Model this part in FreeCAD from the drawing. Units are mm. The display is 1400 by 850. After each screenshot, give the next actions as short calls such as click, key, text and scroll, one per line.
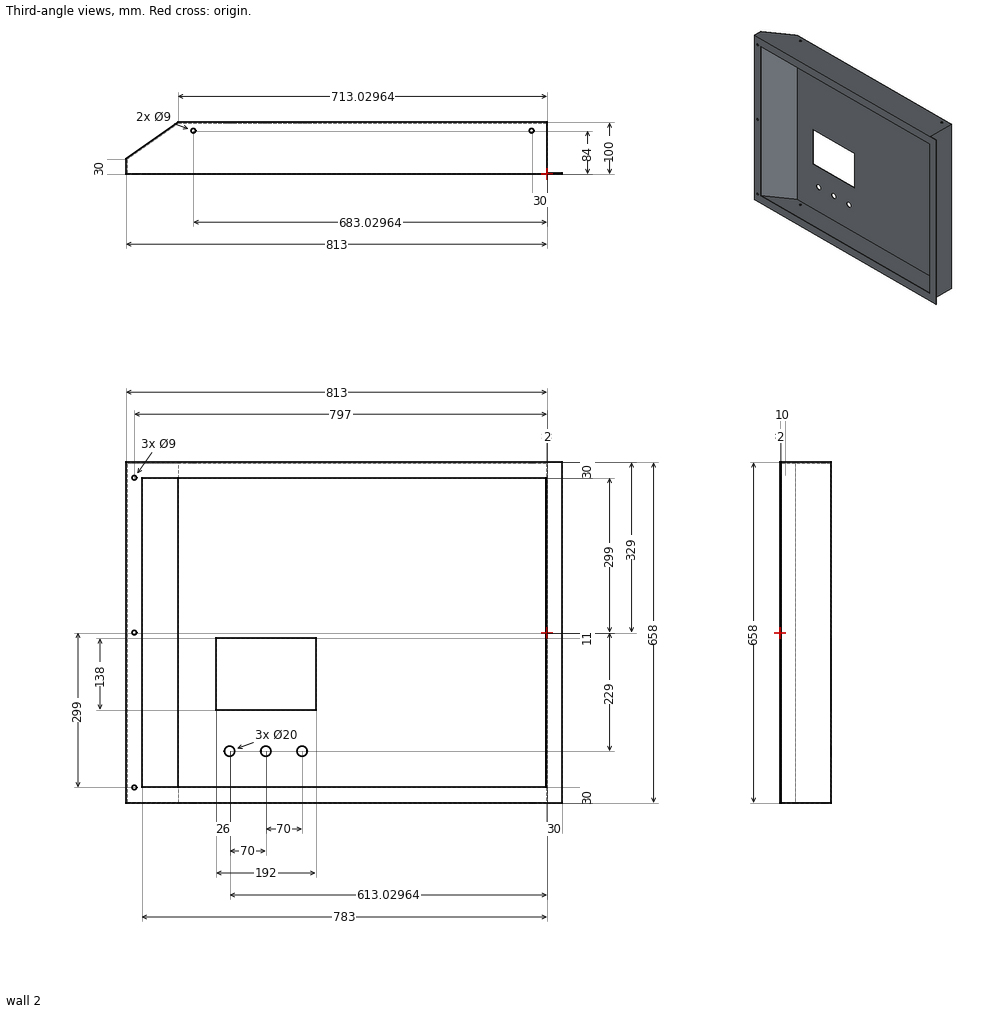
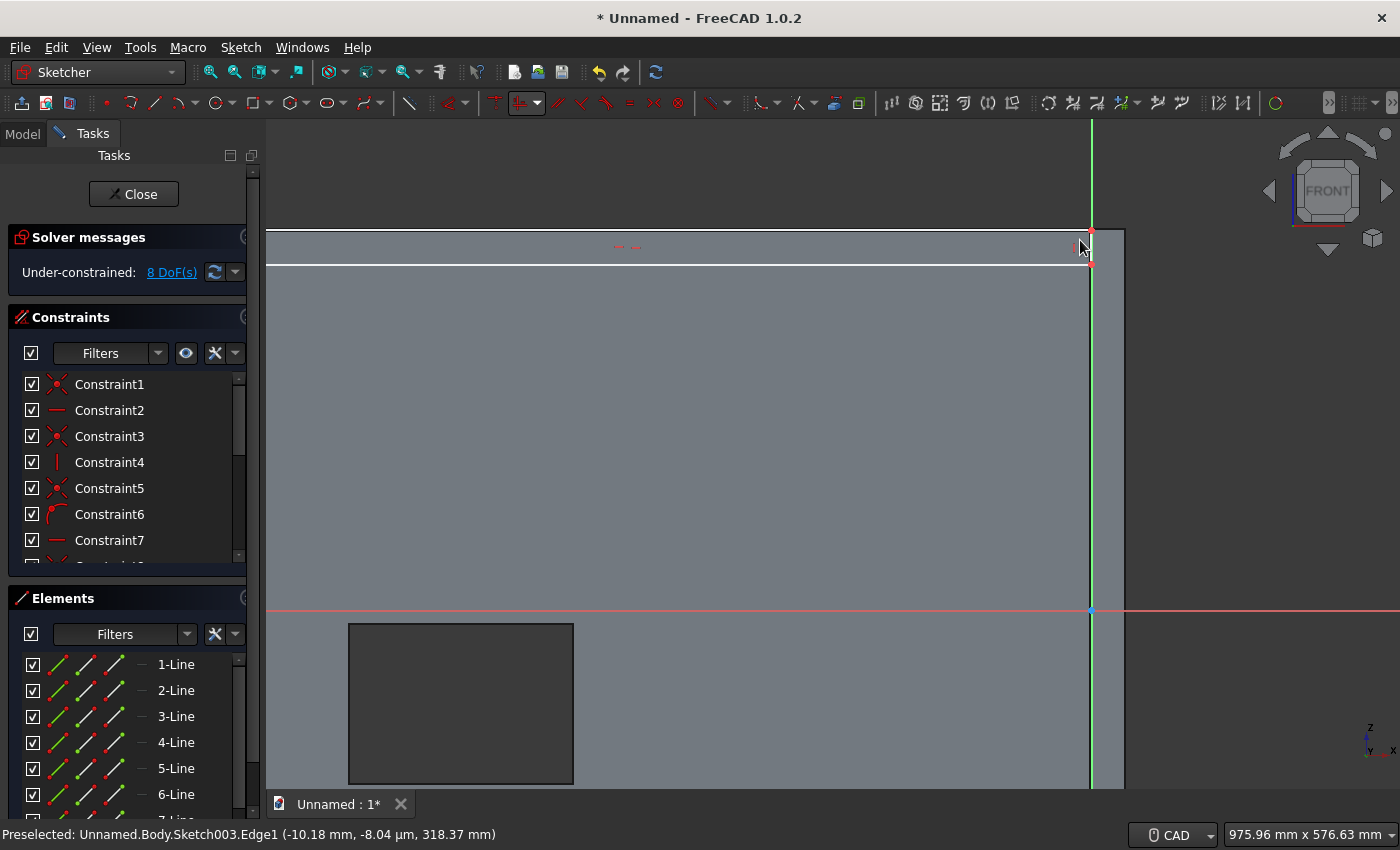
scroll(941, 263, down, 3)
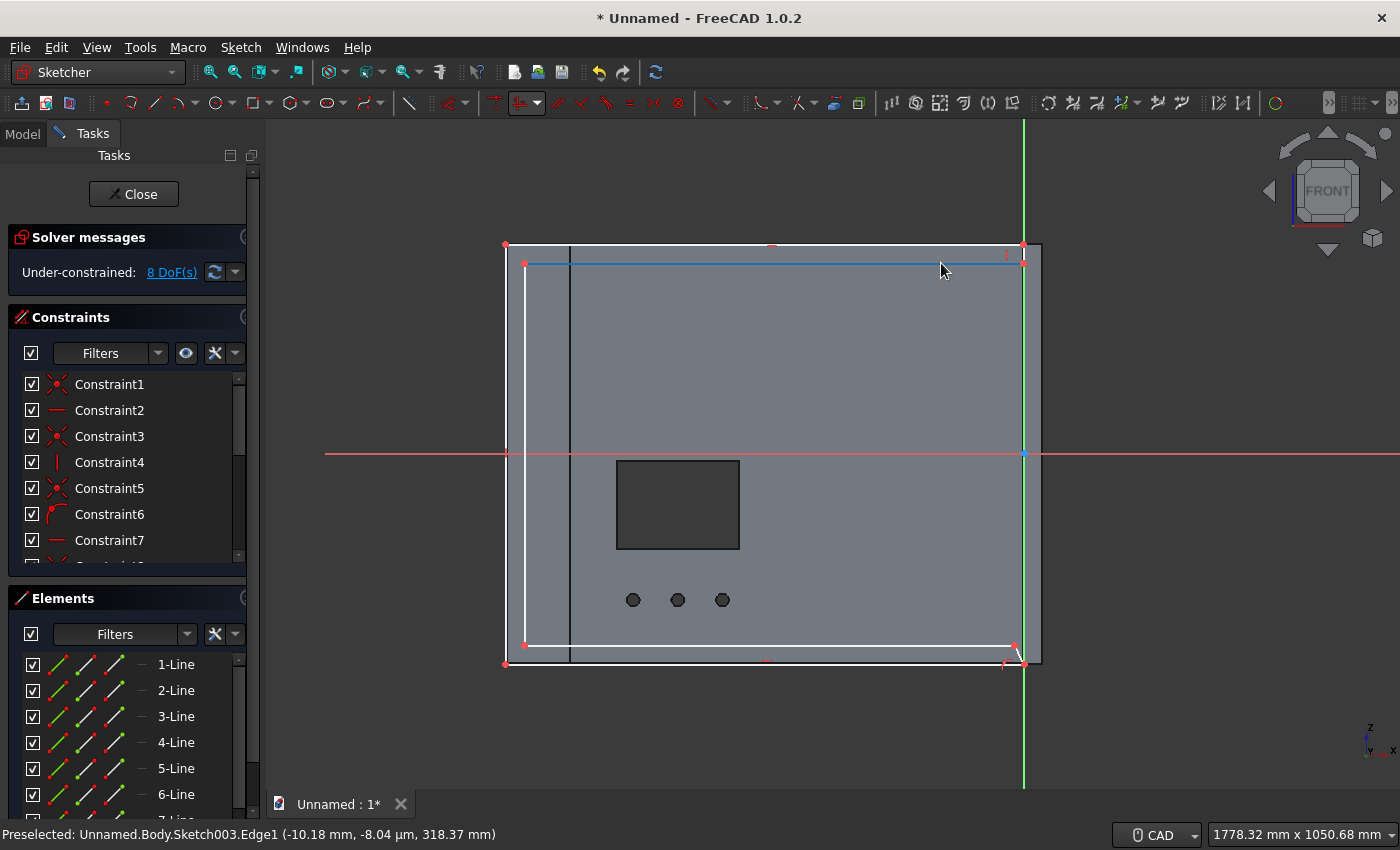
scroll(1018, 652, up, 4)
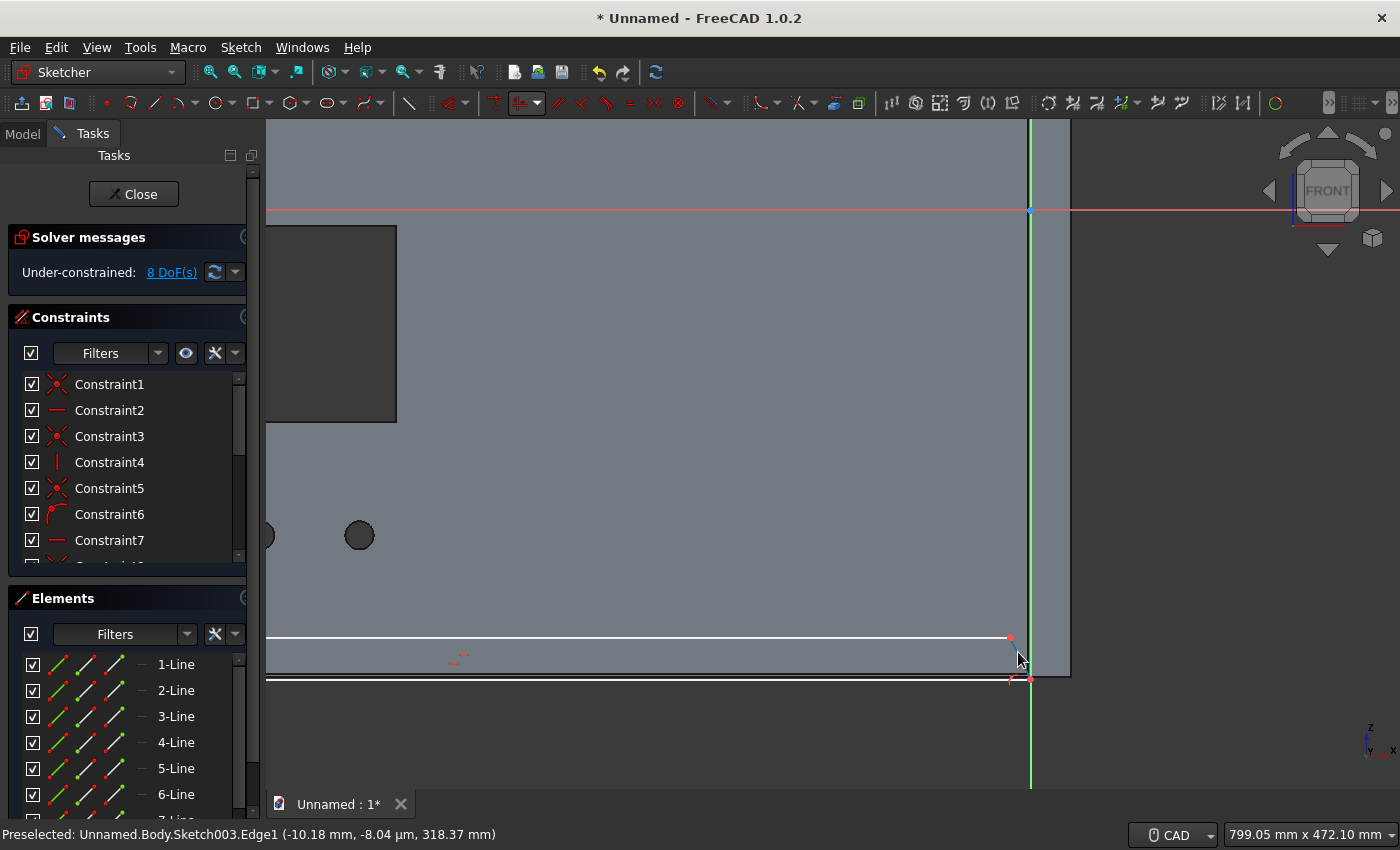
click(1016, 650)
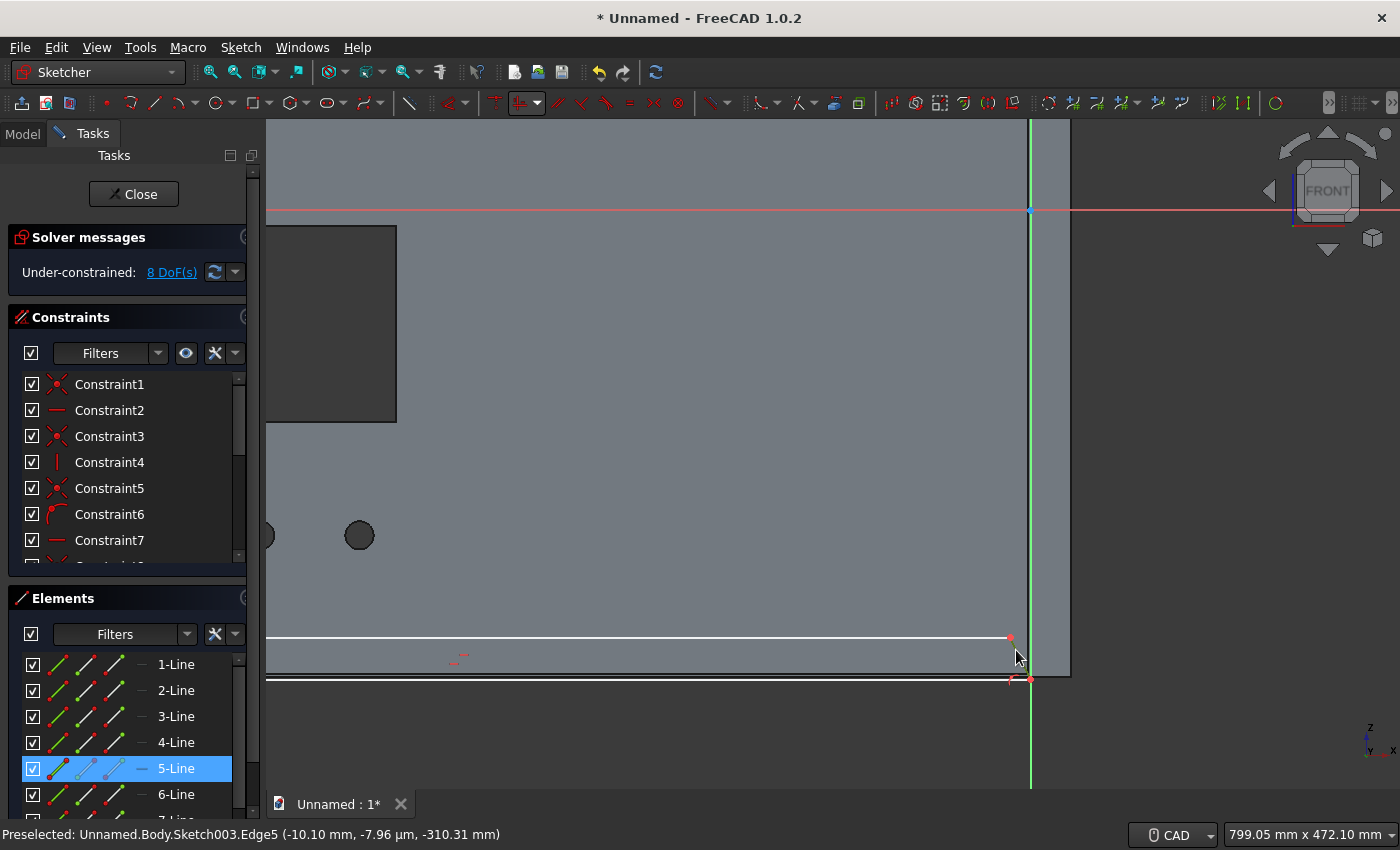
key(v)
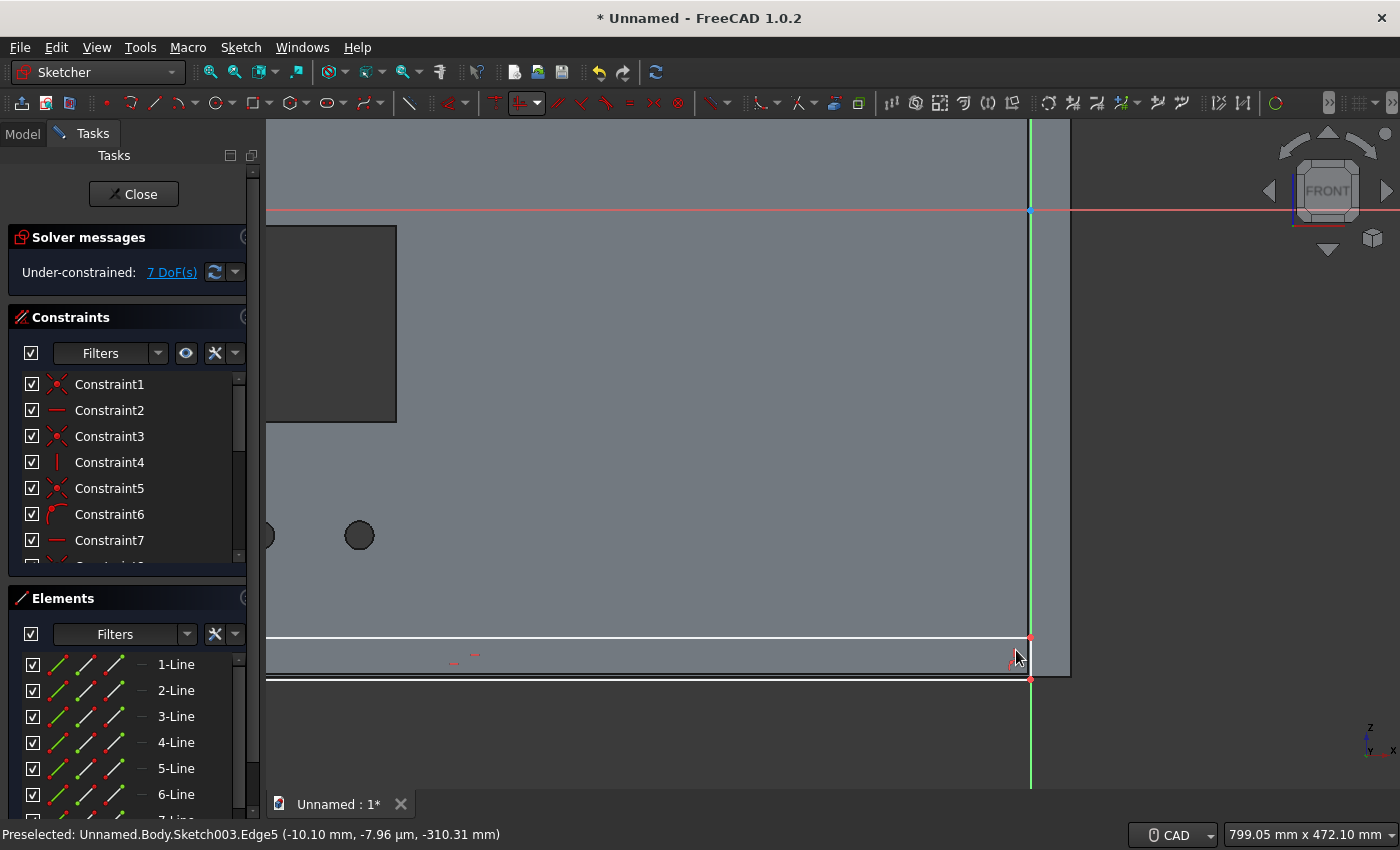
scroll(1018, 653, down, 4)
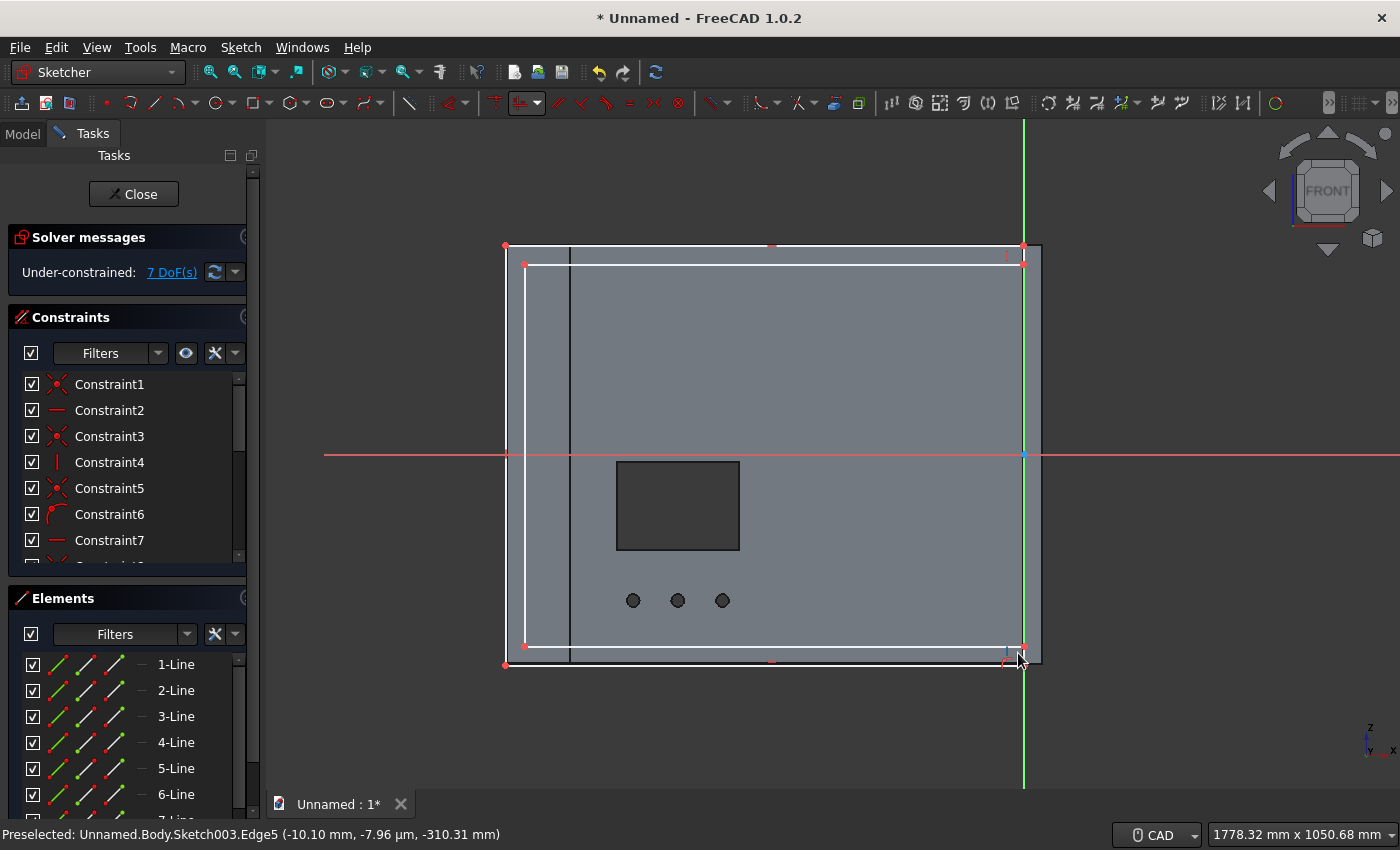
click(1024, 265)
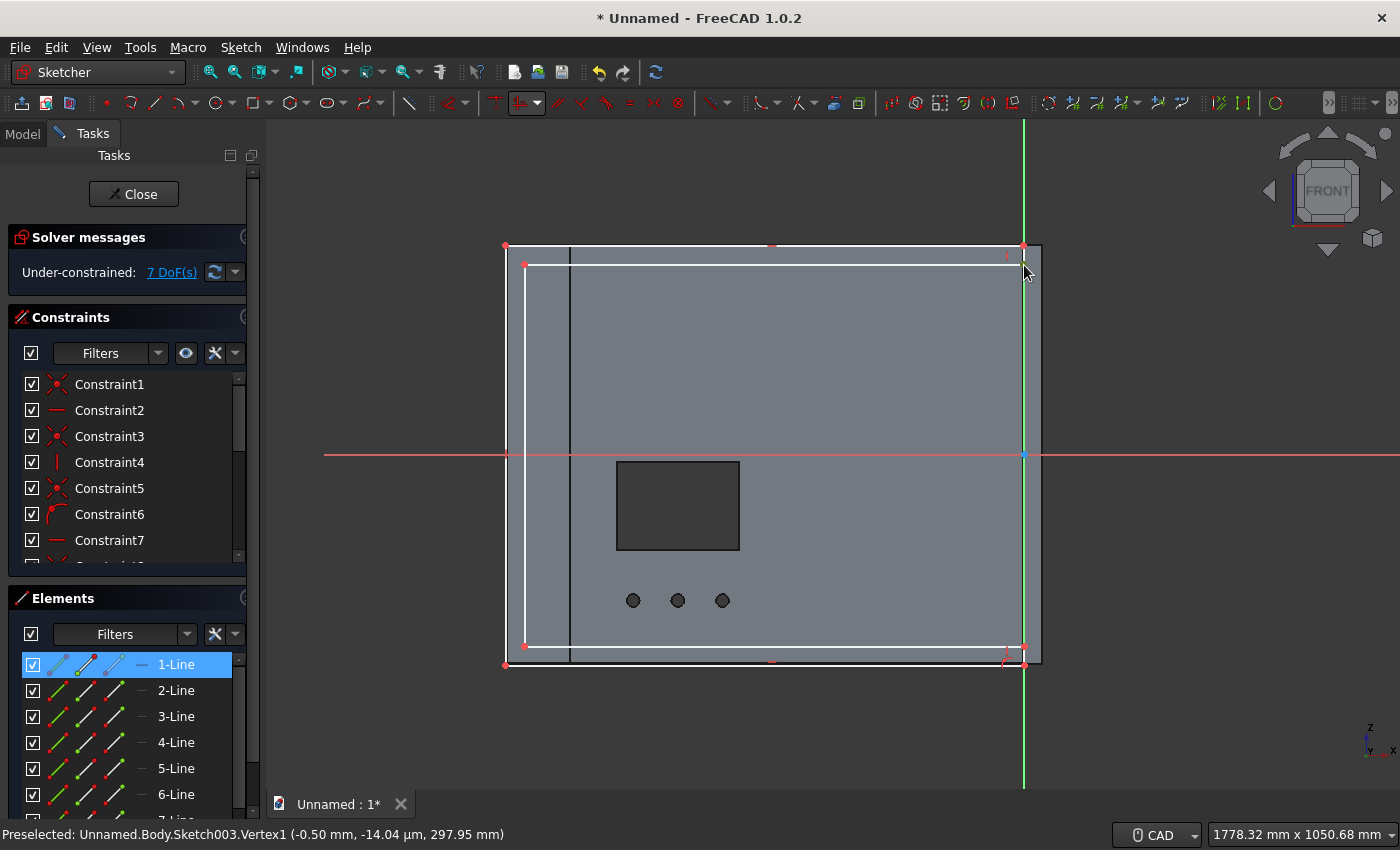
click(1024, 717)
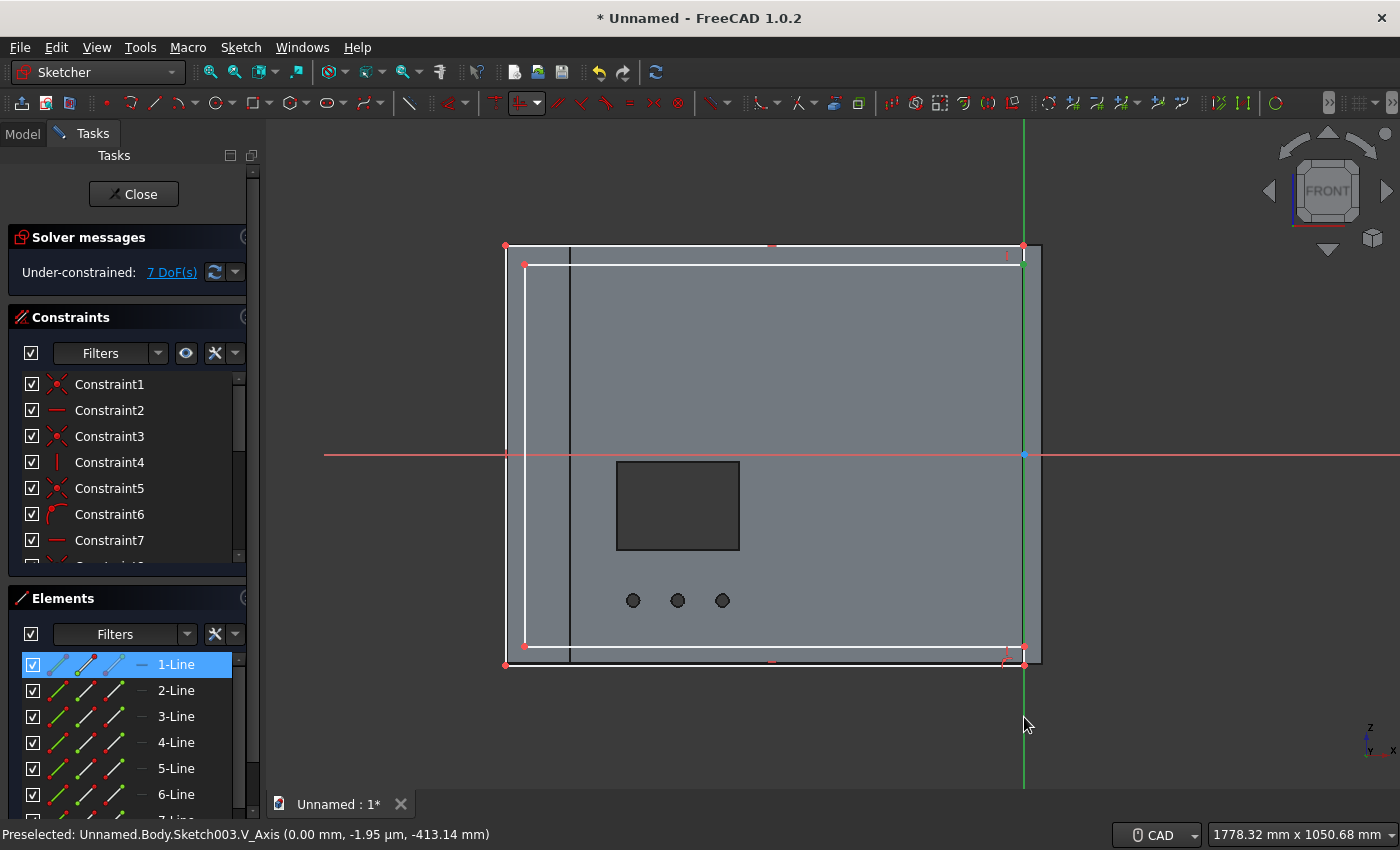
click(496, 104)